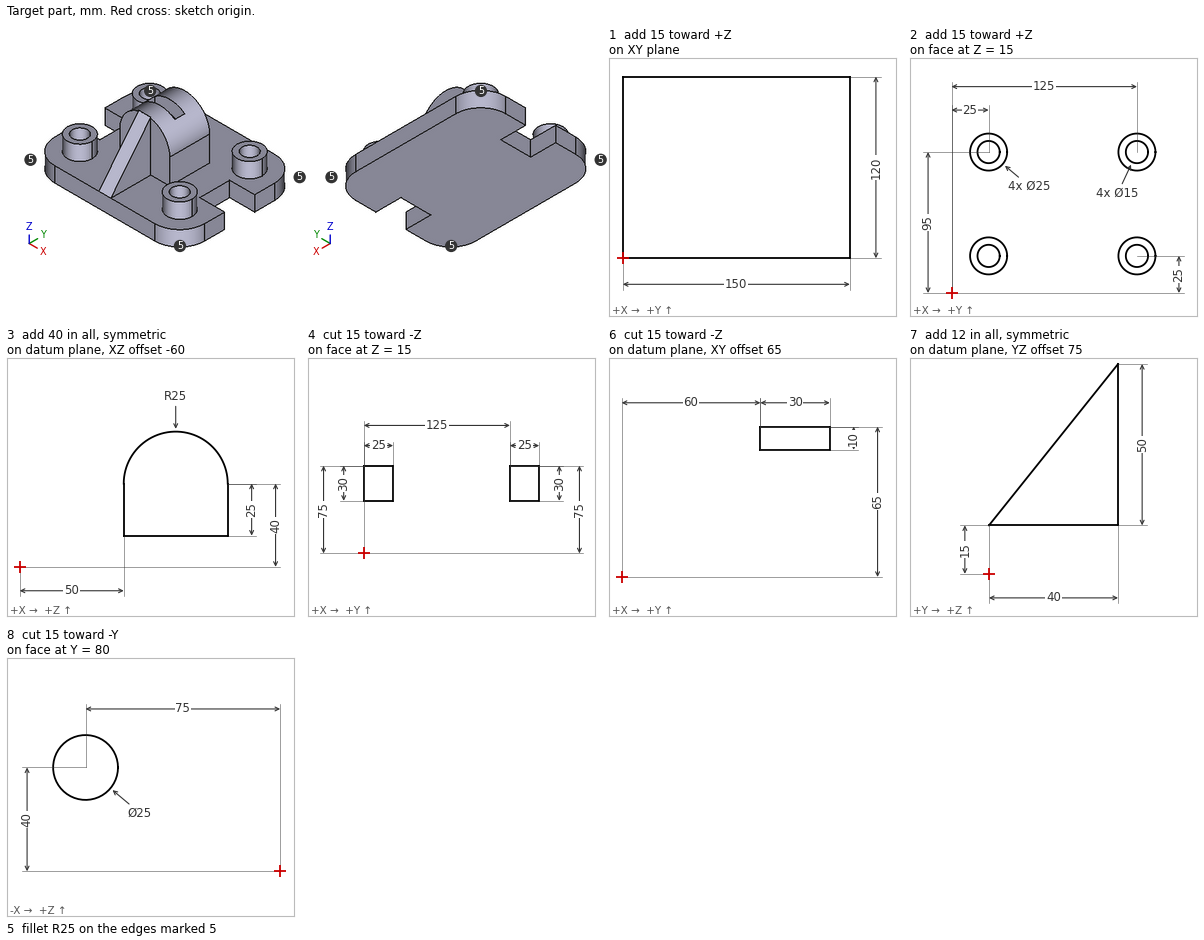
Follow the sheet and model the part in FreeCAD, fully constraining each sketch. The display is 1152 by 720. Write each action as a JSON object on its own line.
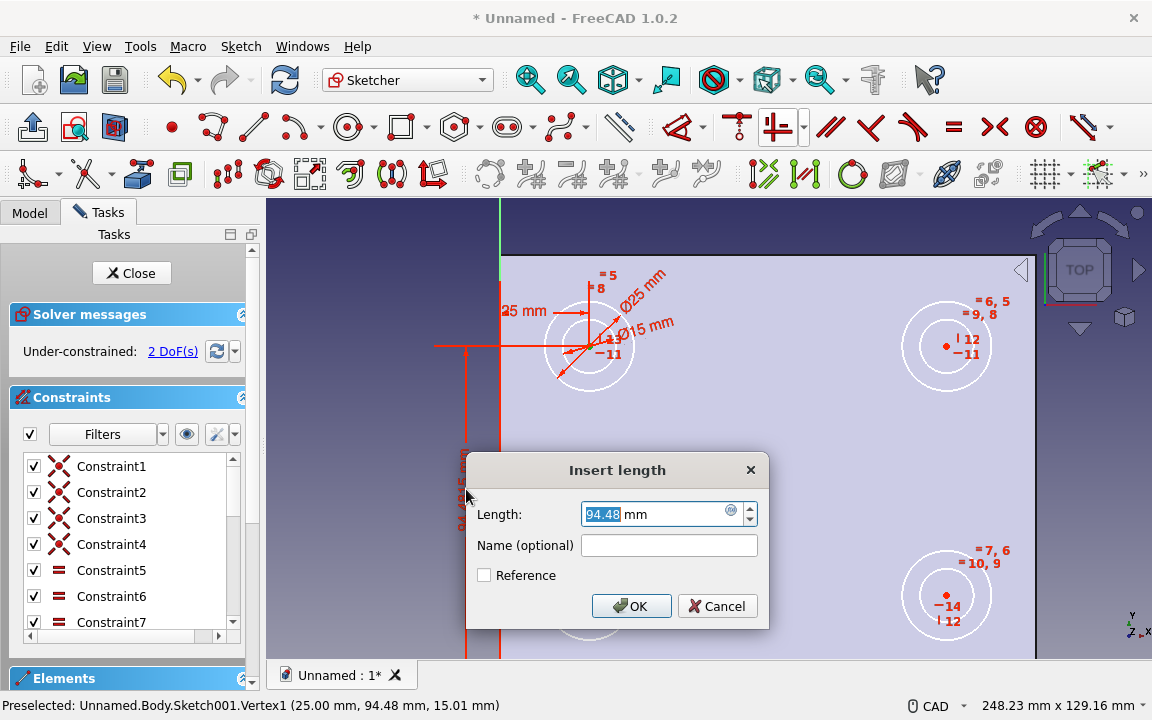
{"action": "type", "text": "95"}
{"action": "key", "text": "Return"}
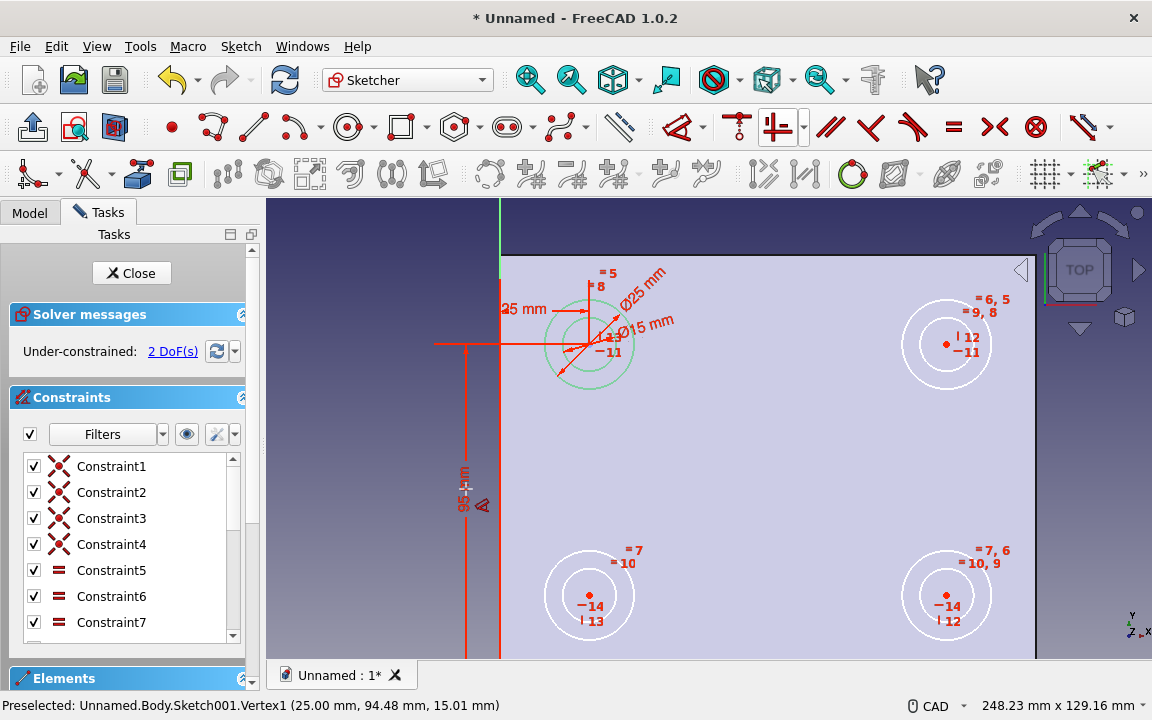
{"action": "left_click", "coordinate": [947, 595]}
{"action": "left_click", "coordinate": [466, 613]}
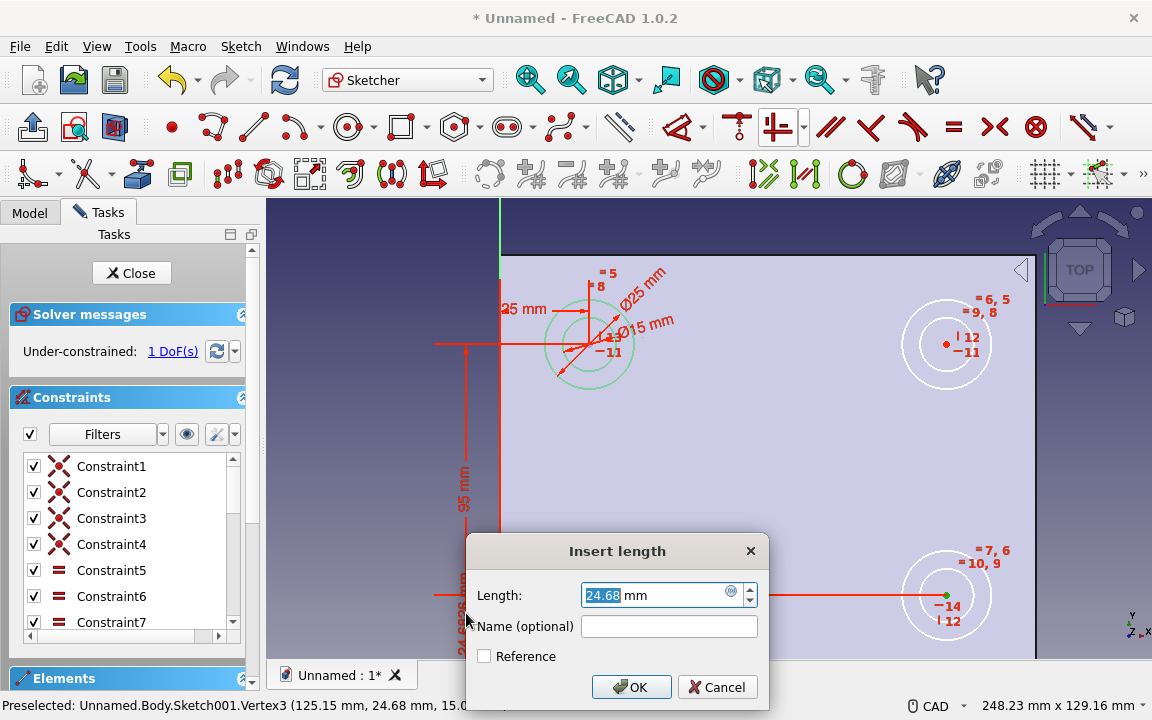
{"action": "type", "text": "25"}
{"action": "key", "text": "Return"}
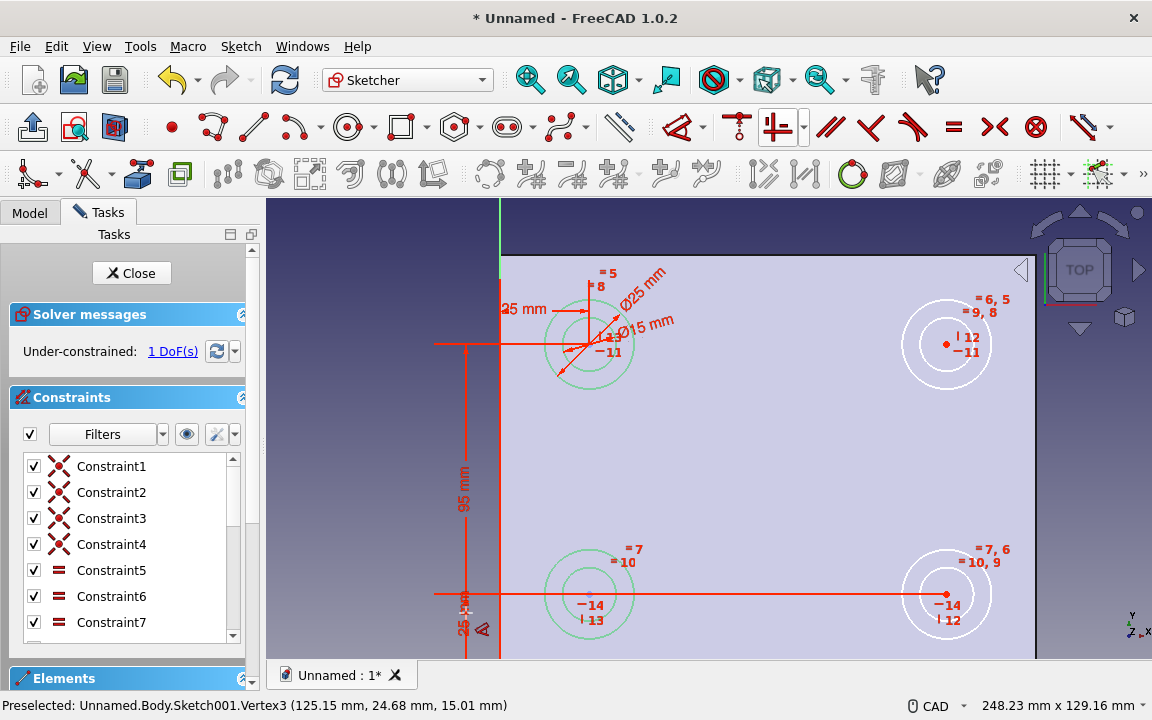
{"action": "left_click", "coordinate": [947, 344]}
{"action": "left_click", "coordinate": [723, 310]}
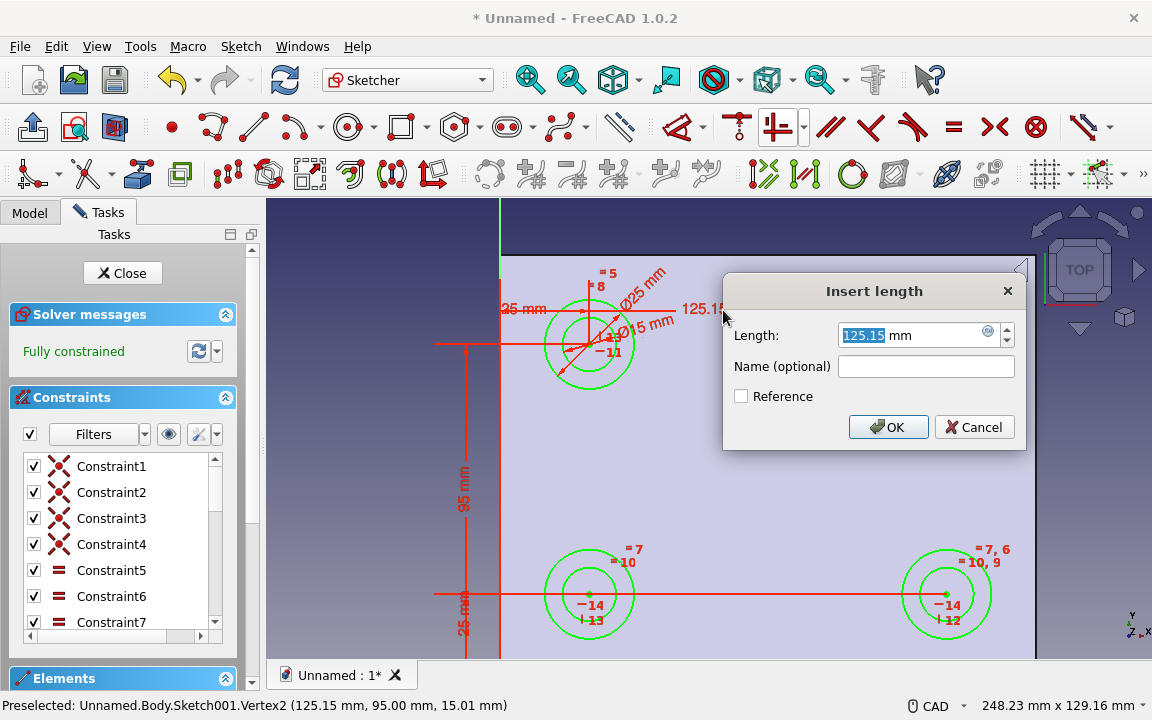
{"action": "type", "text": "125"}
{"action": "key", "text": "Return"}
{"action": "key", "text": "Escape"}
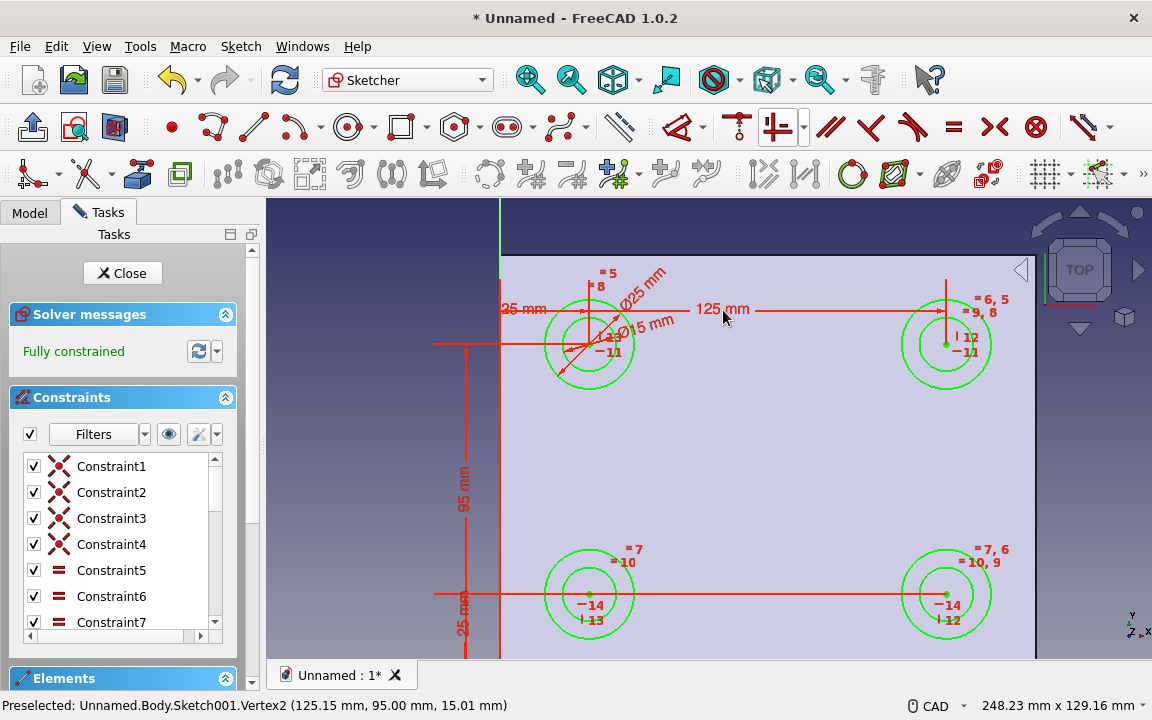
{"action": "left_click", "coordinate": [123, 273]}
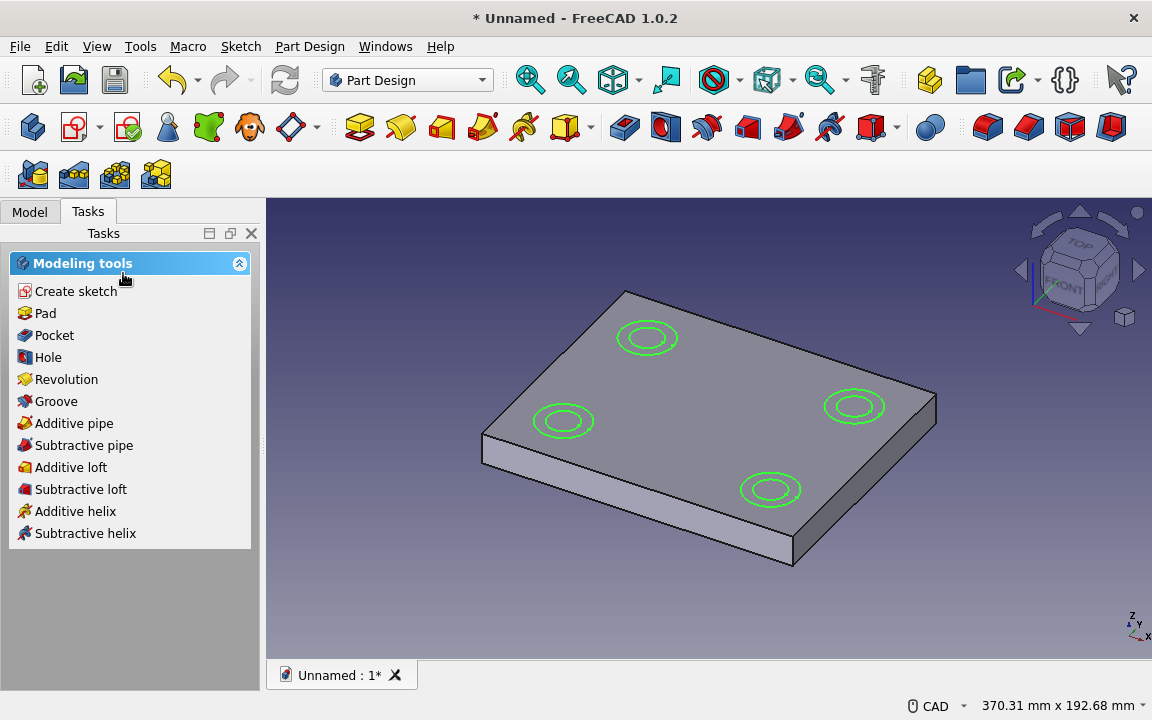
{"action": "left_click", "coordinate": [360, 128]}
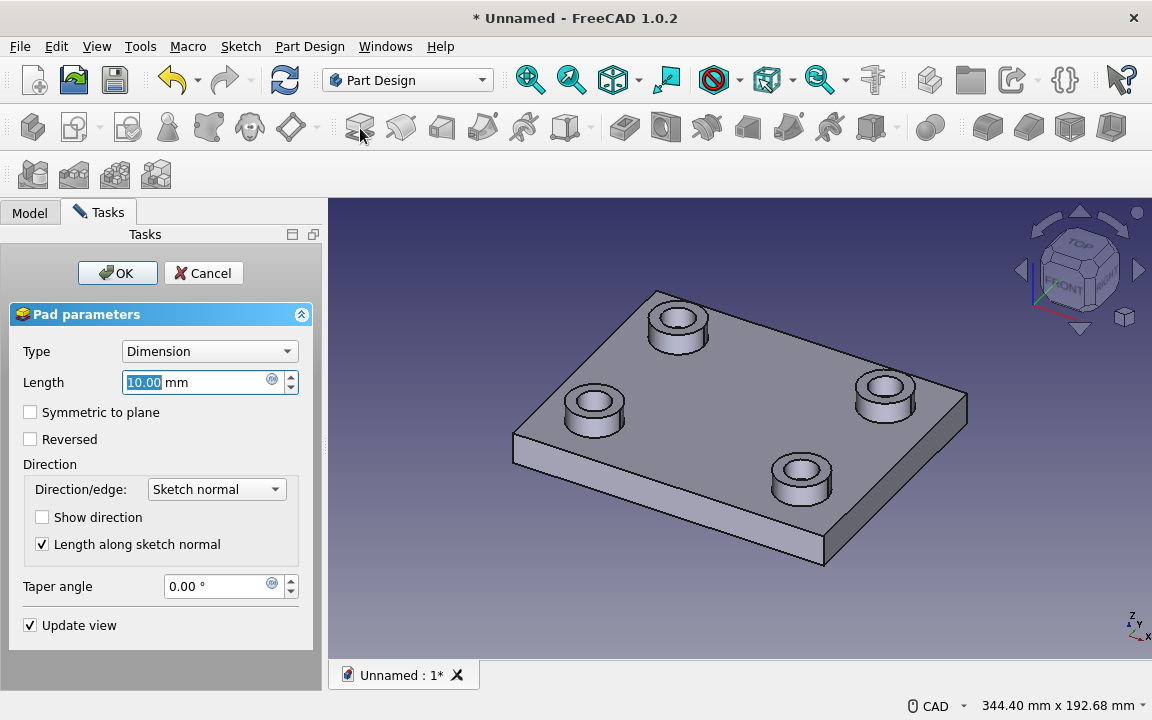
{"action": "type", "text": "15"}
{"action": "key", "text": "Tab"}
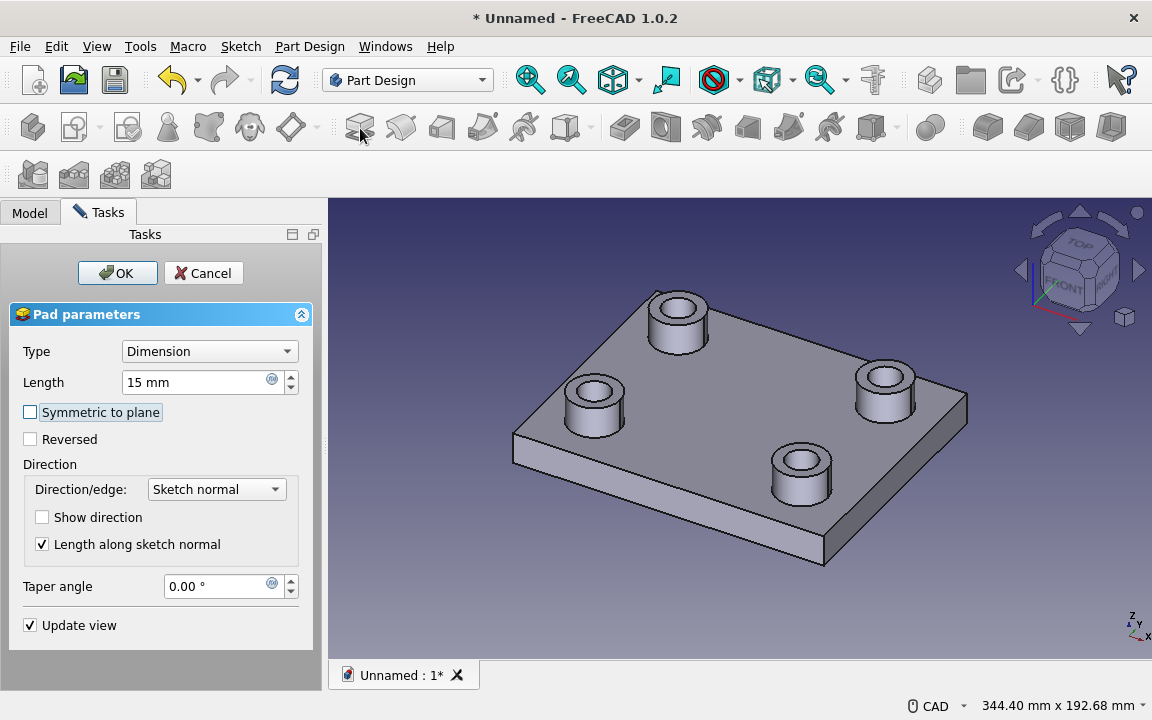
{"action": "left_click", "coordinate": [118, 273]}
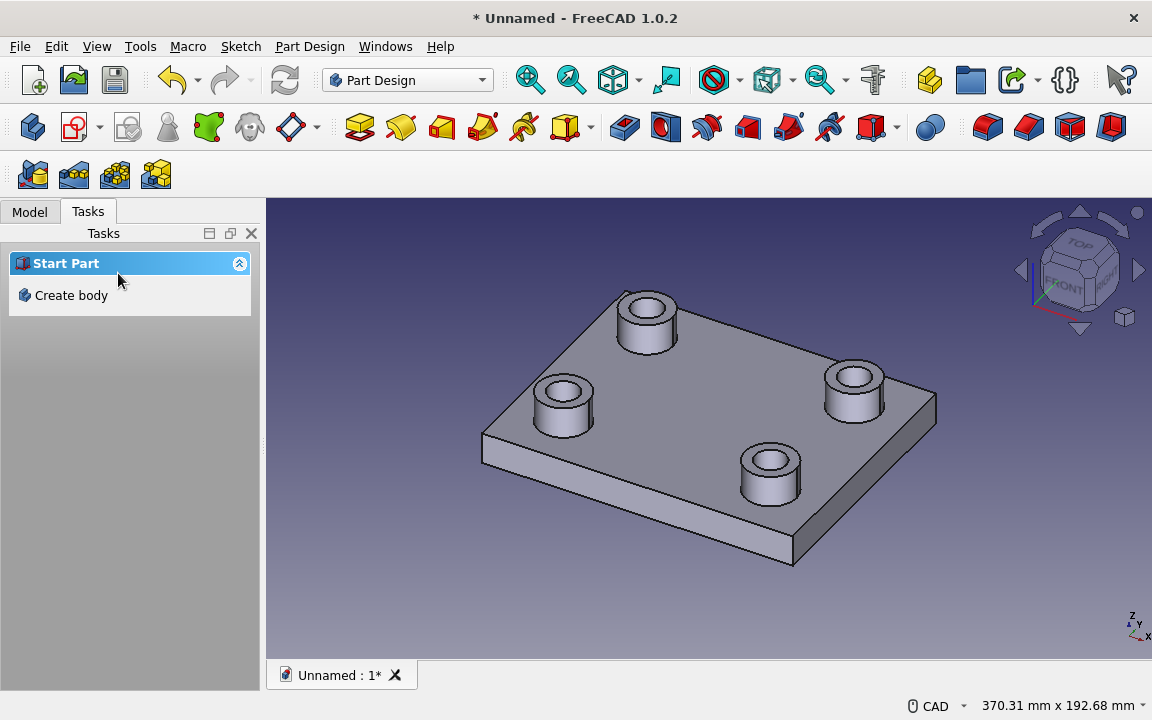
{"action": "left_click", "coordinate": [30, 212]}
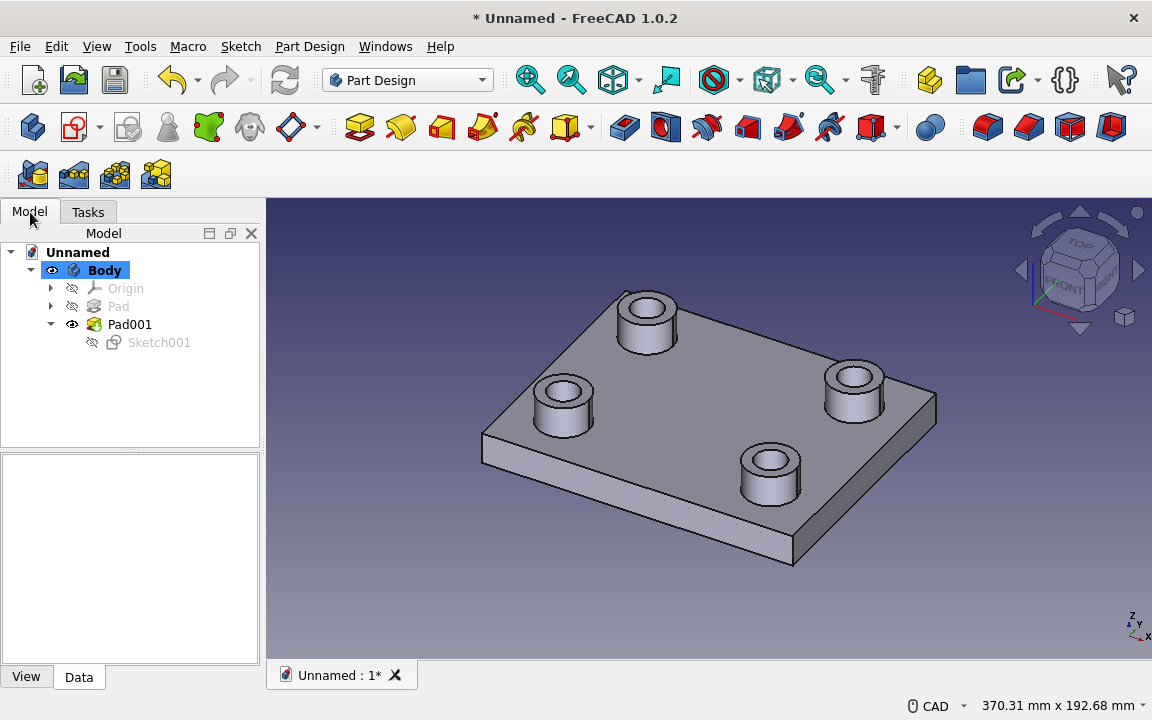
{"action": "left_click", "coordinate": [51, 288]}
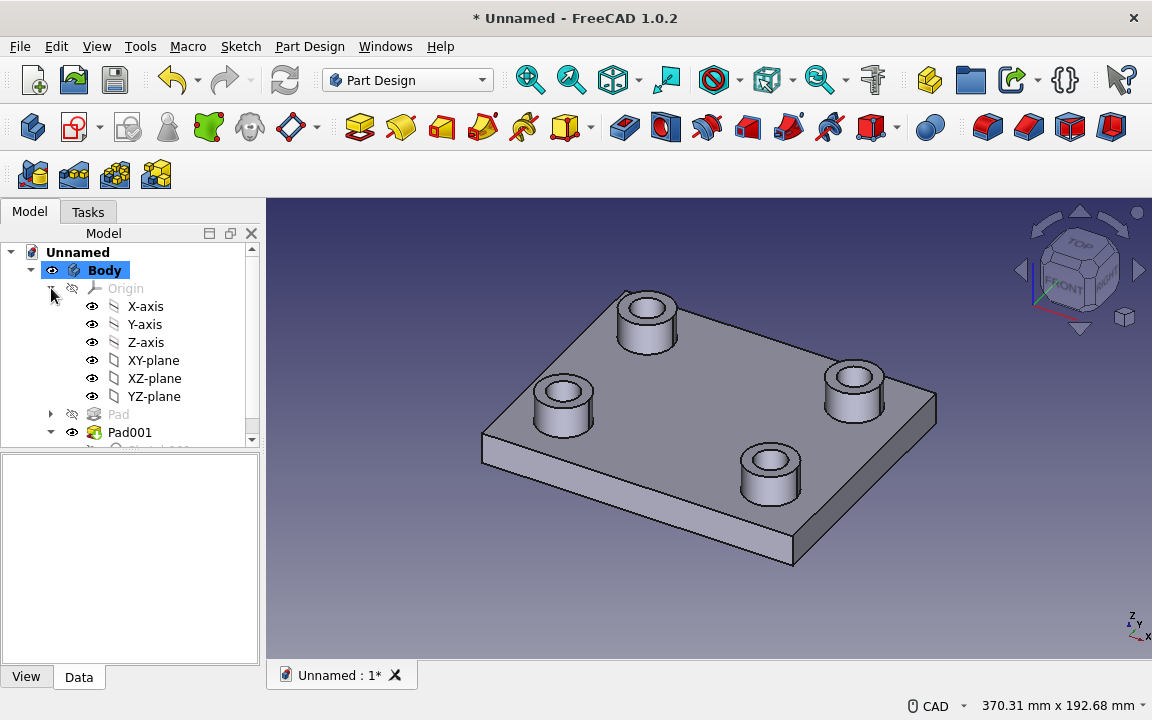
{"action": "left_click", "coordinate": [137, 378]}